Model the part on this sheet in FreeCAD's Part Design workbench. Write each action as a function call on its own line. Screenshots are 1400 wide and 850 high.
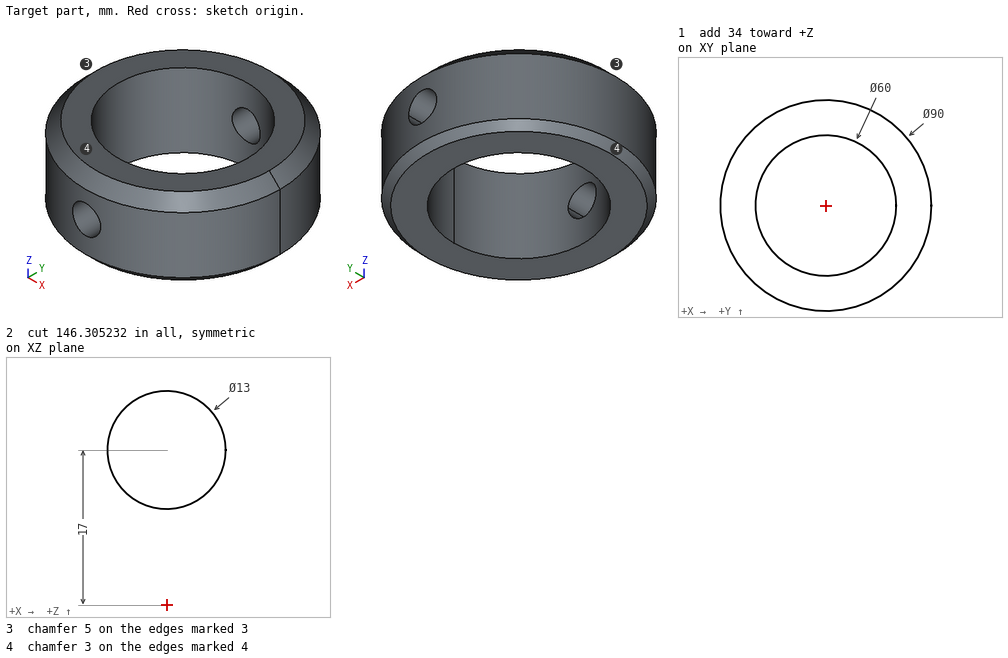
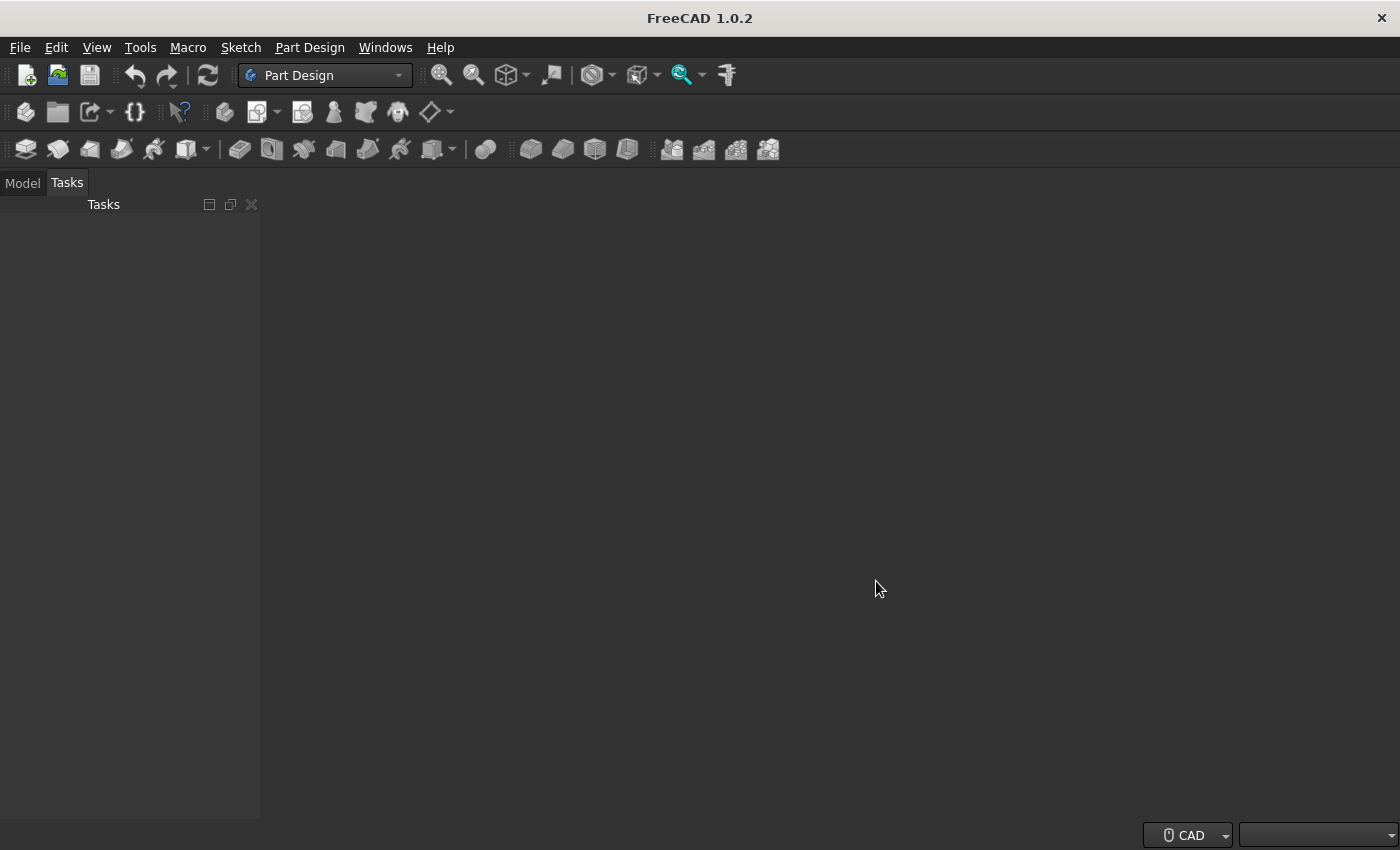
key(ctrl+n)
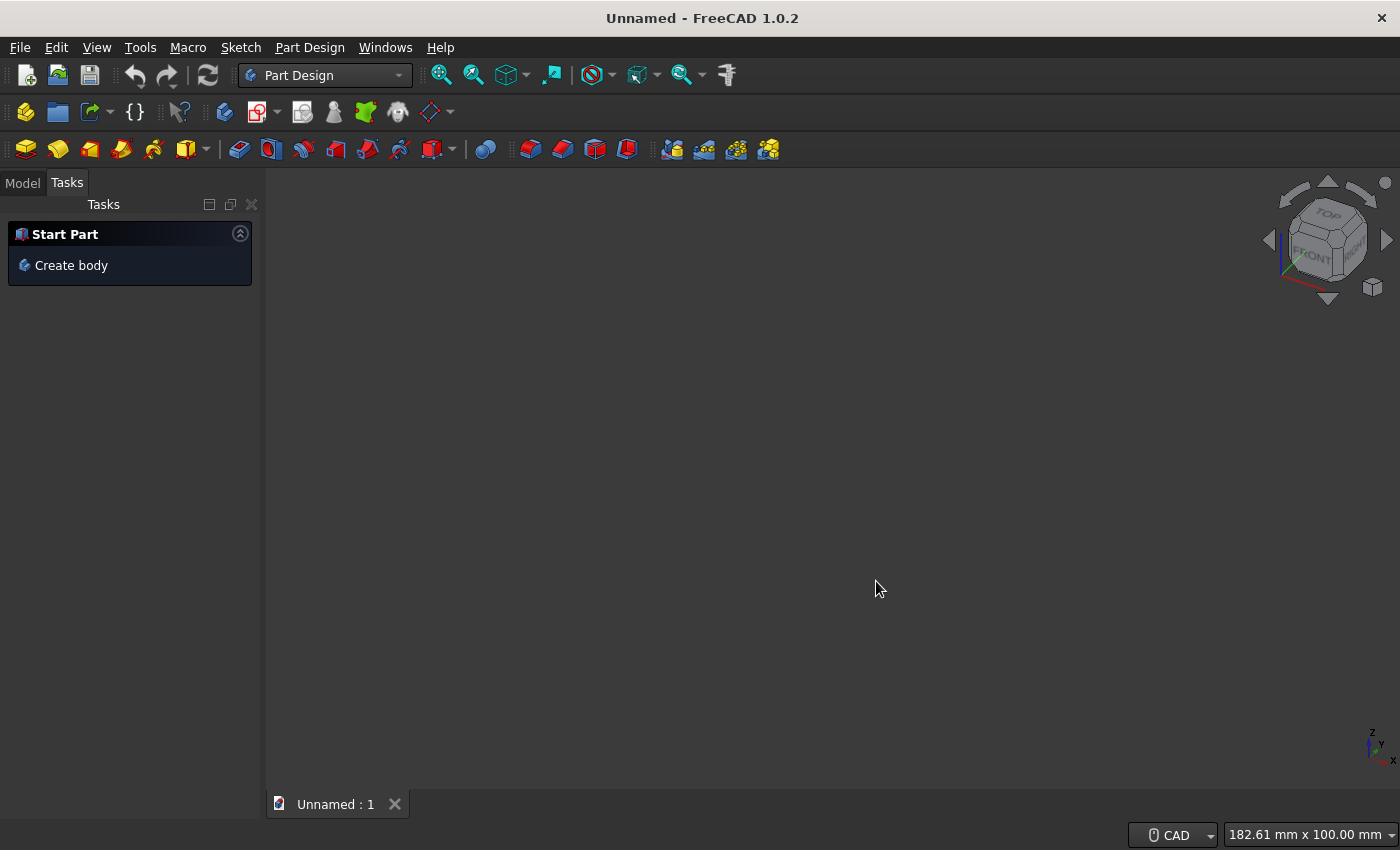
click(258, 112)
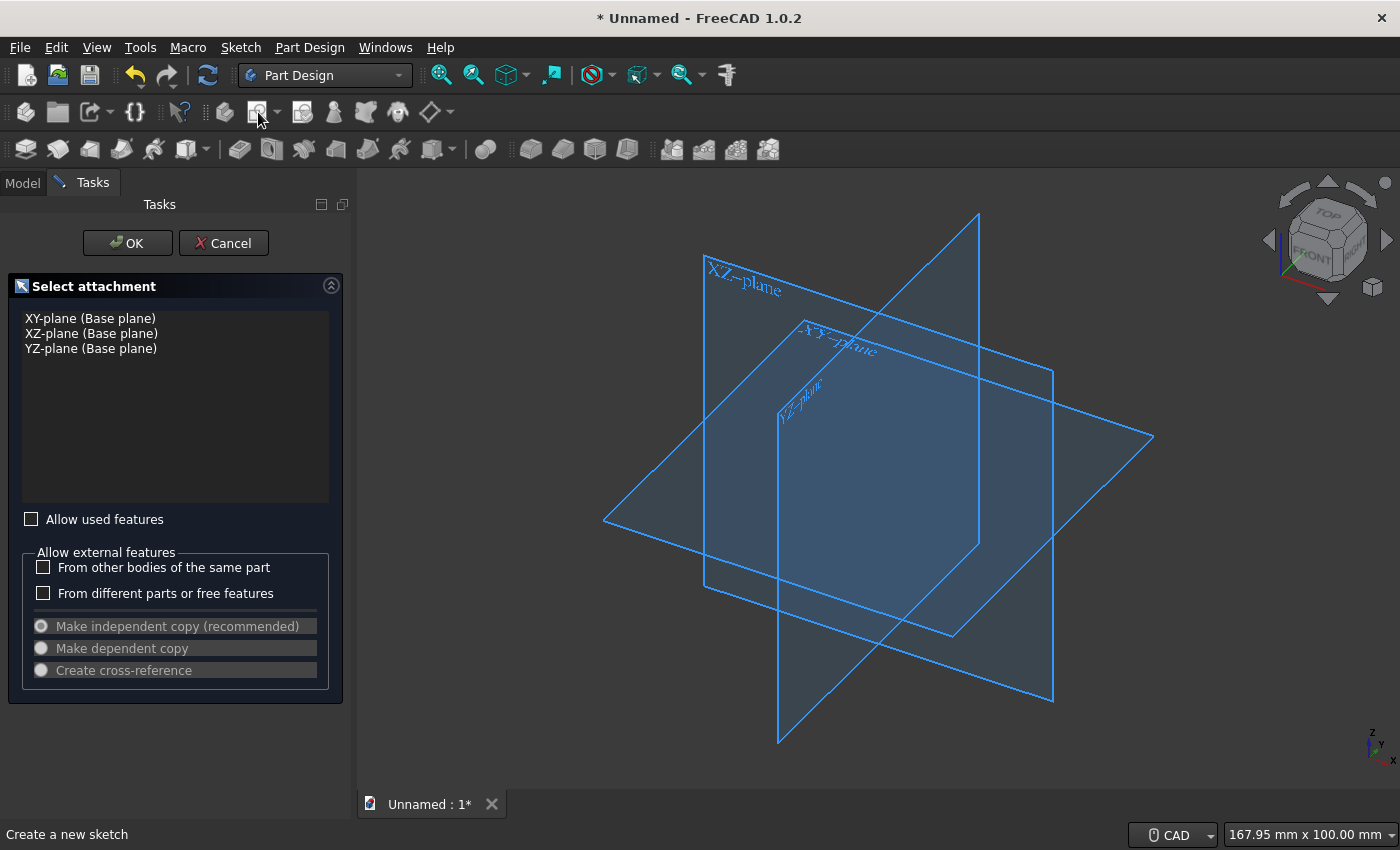
click(82, 318)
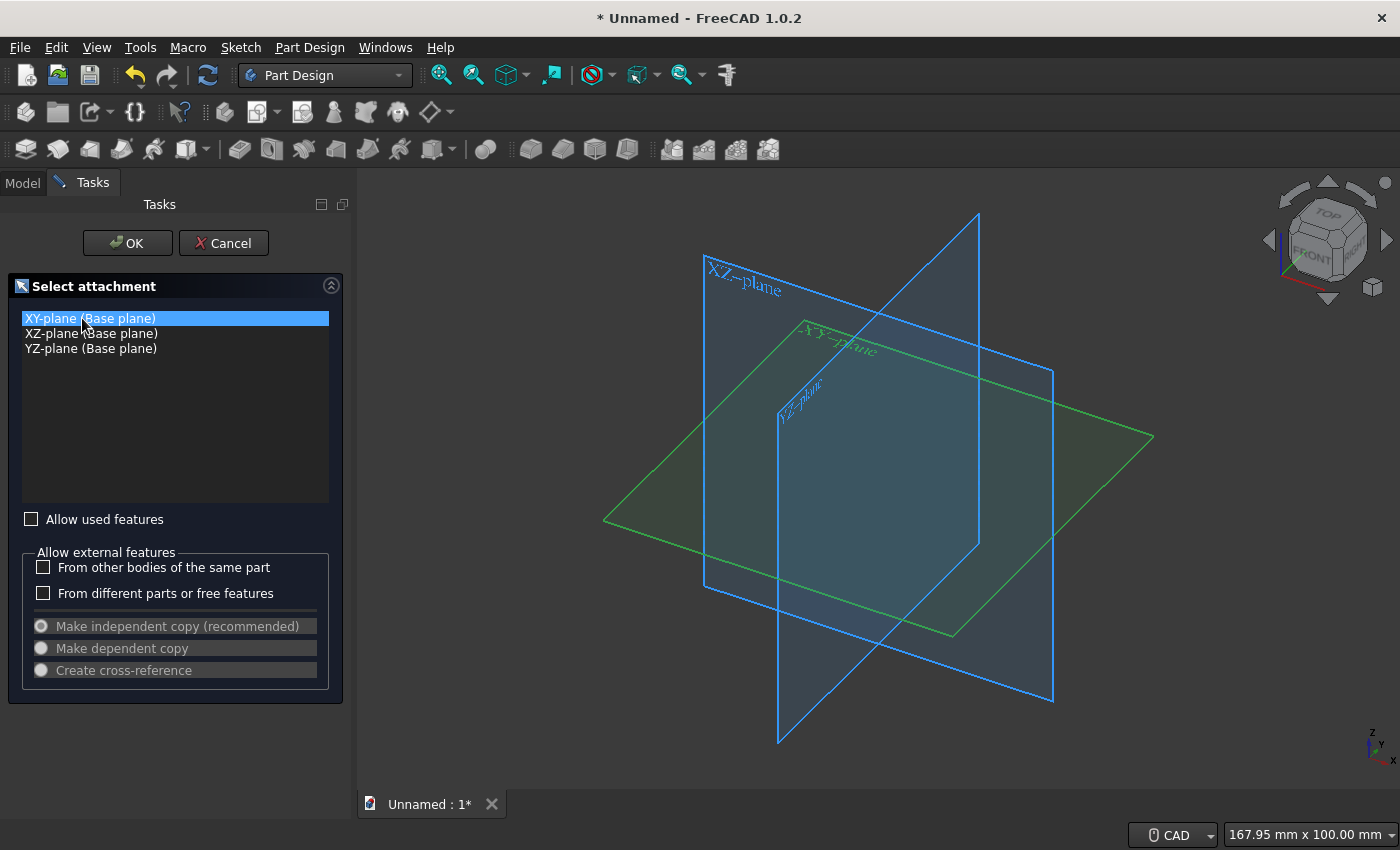
click(128, 243)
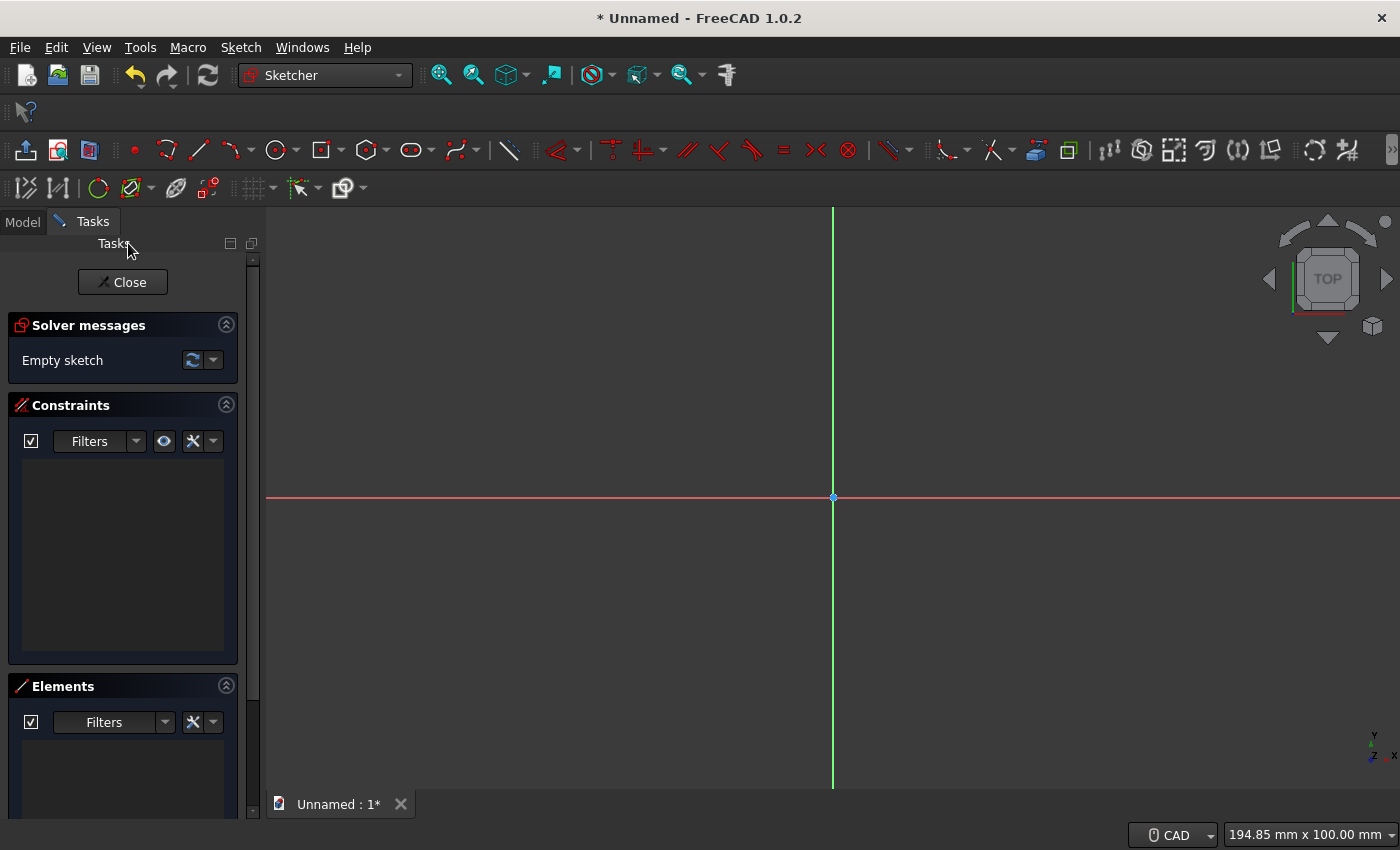
scroll(625, 498, down, 2)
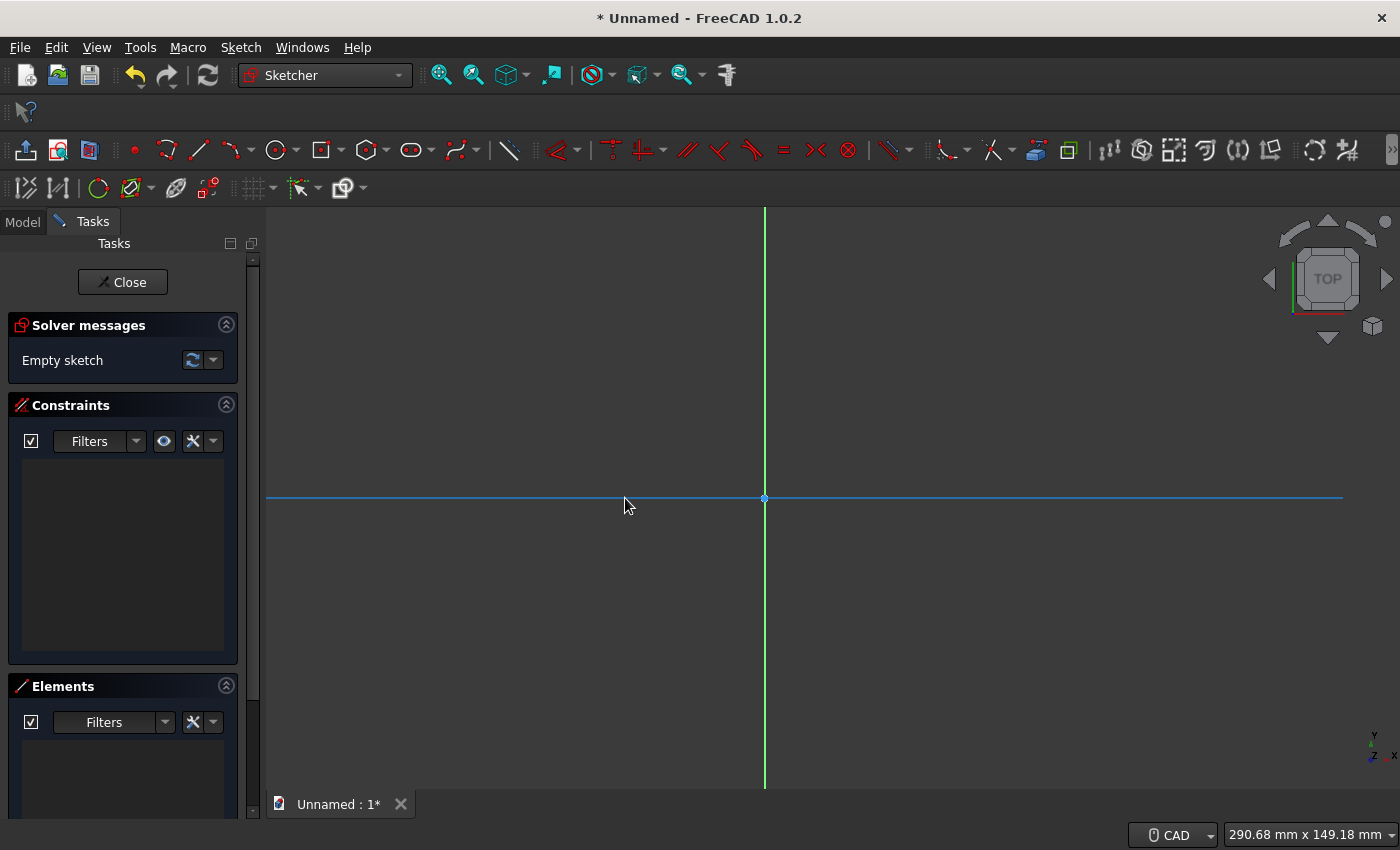
key(g)
key(c)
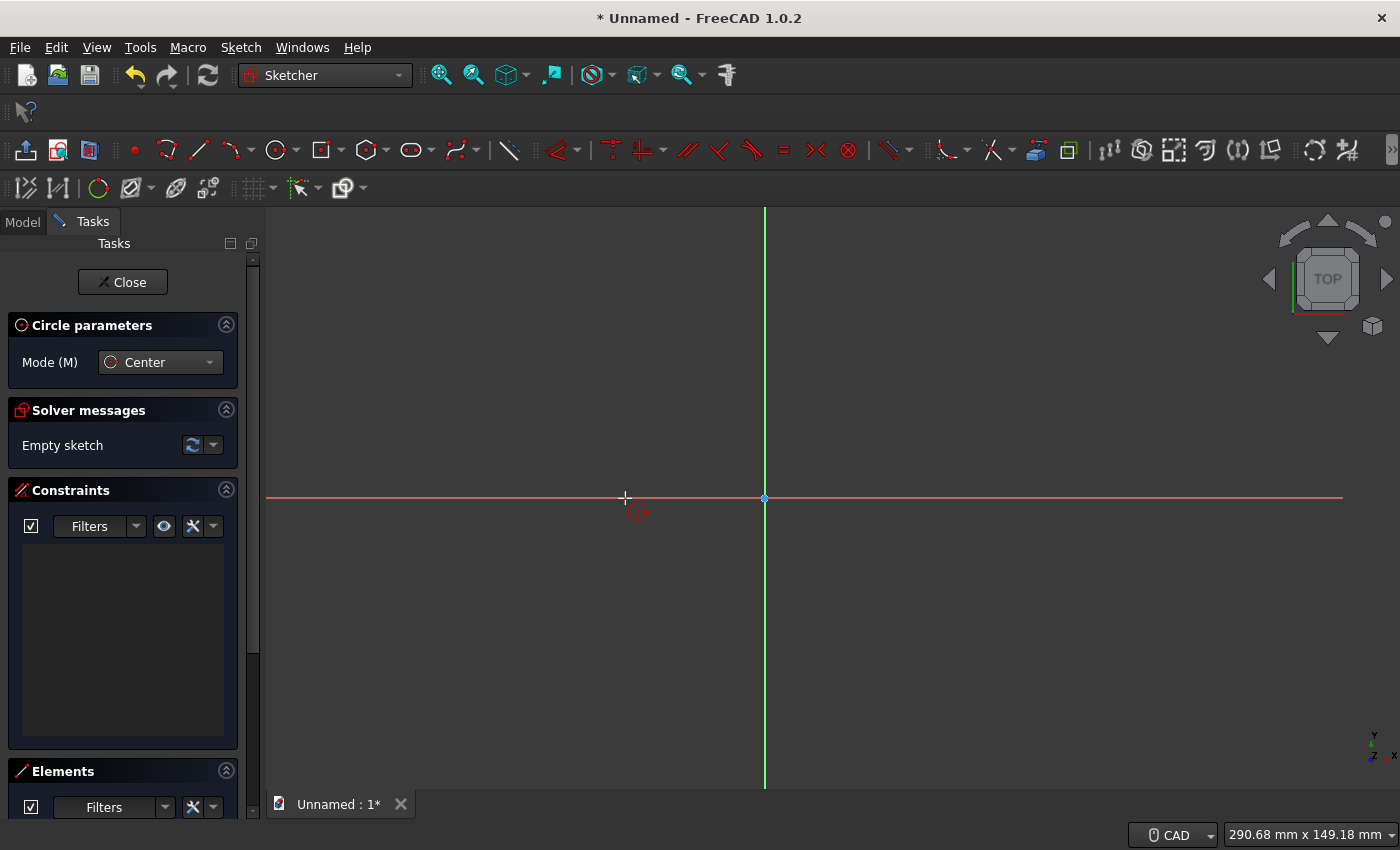
click(765, 498)
click(889, 374)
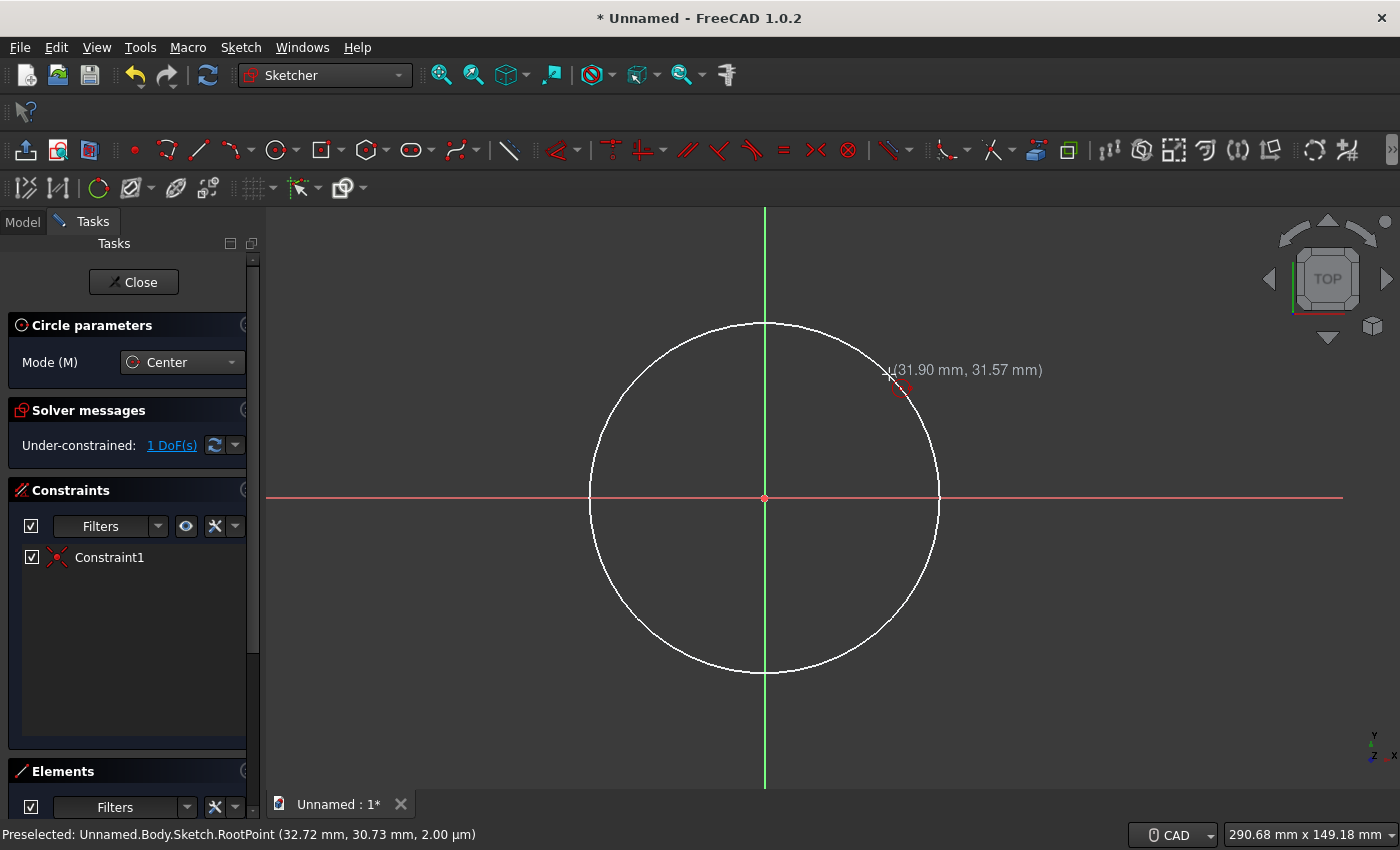
click(765, 498)
click(847, 415)
key(Escape)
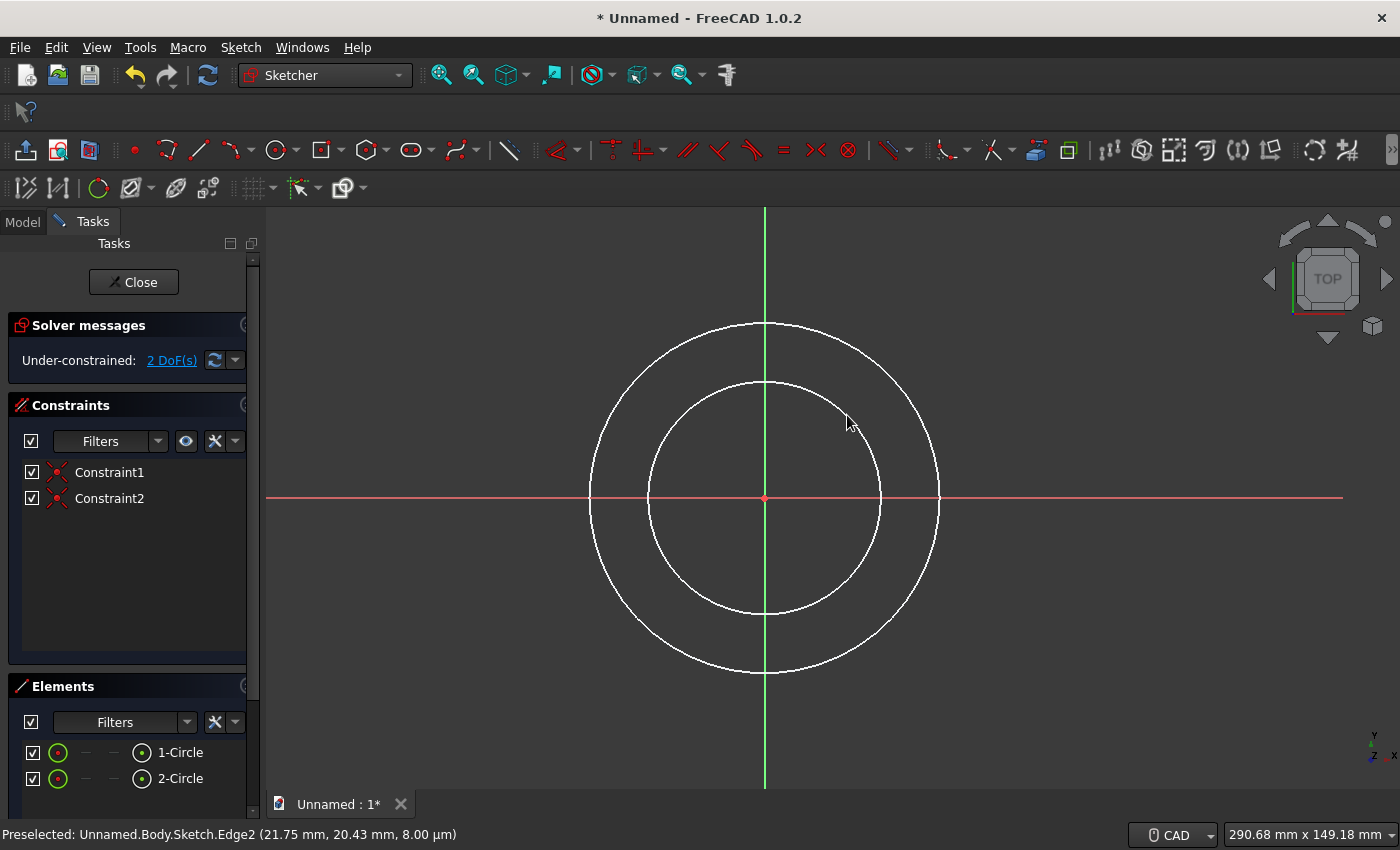
click(556, 150)